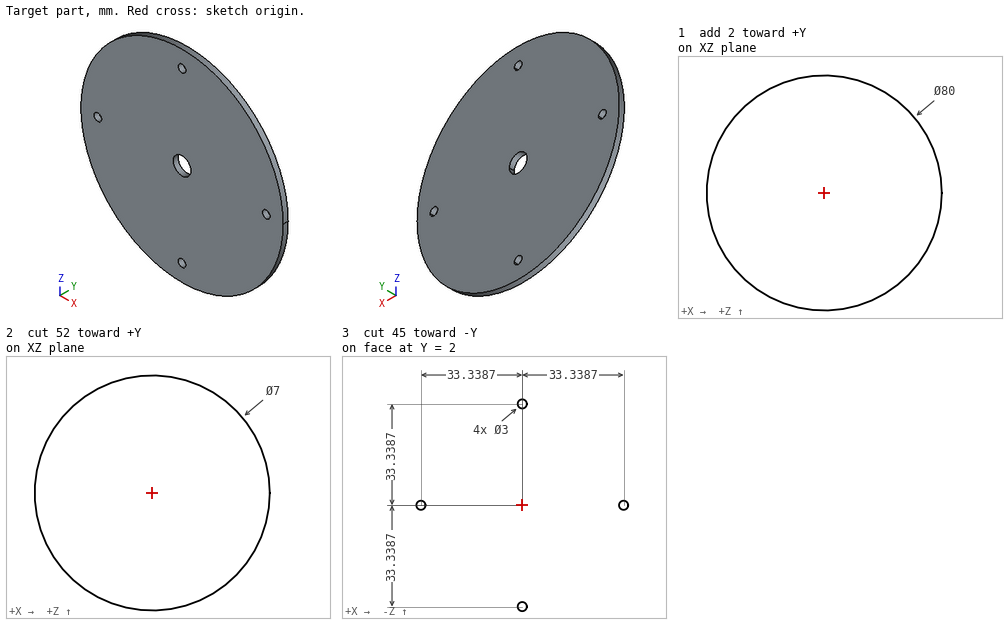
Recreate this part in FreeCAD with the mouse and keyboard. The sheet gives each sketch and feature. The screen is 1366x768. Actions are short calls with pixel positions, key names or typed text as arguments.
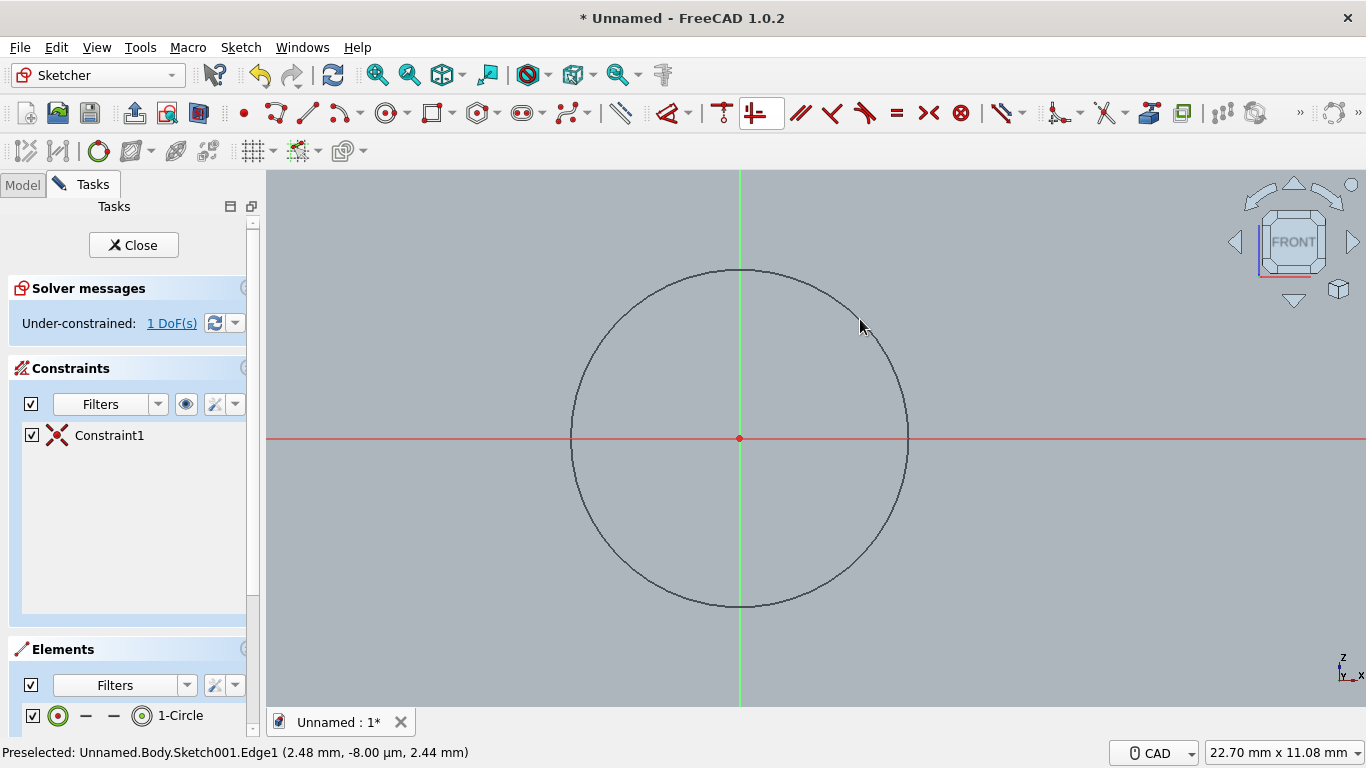
key(d)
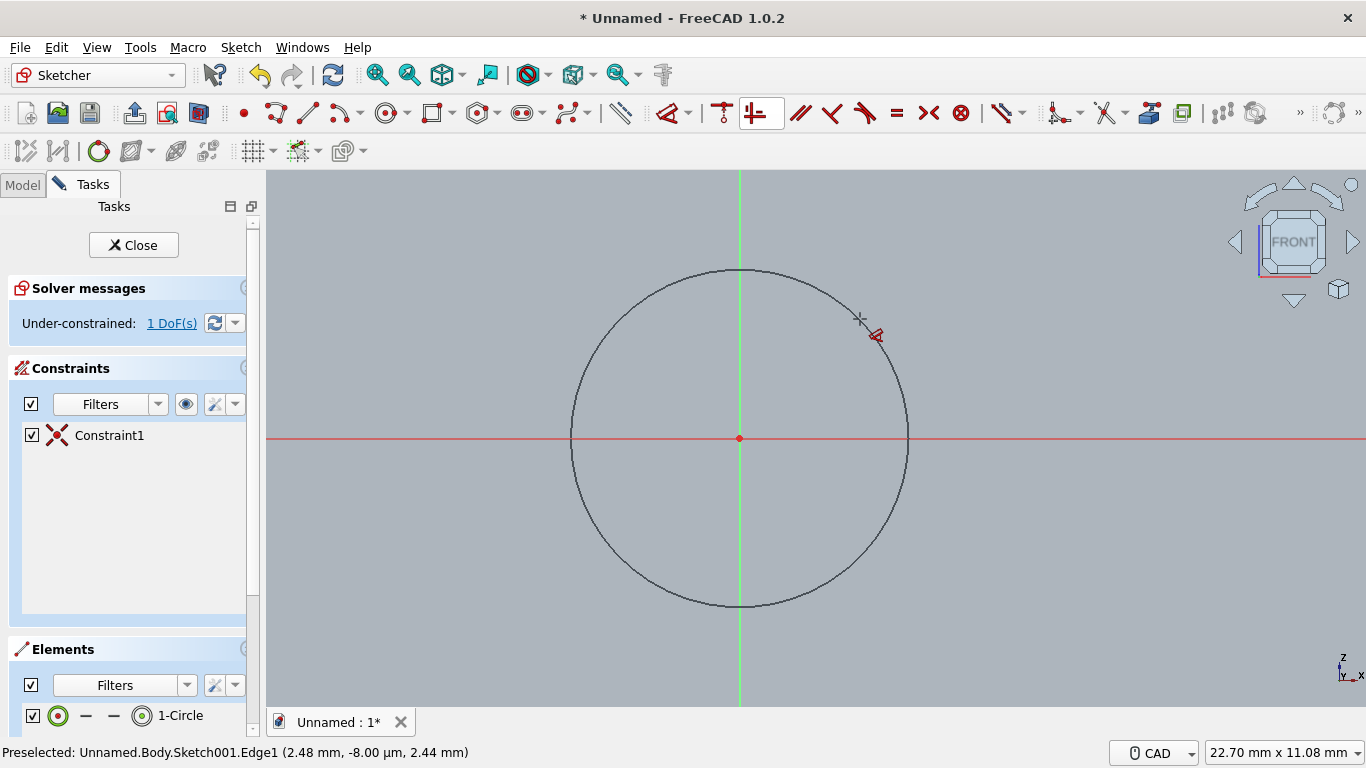
click(859, 319)
click(882, 296)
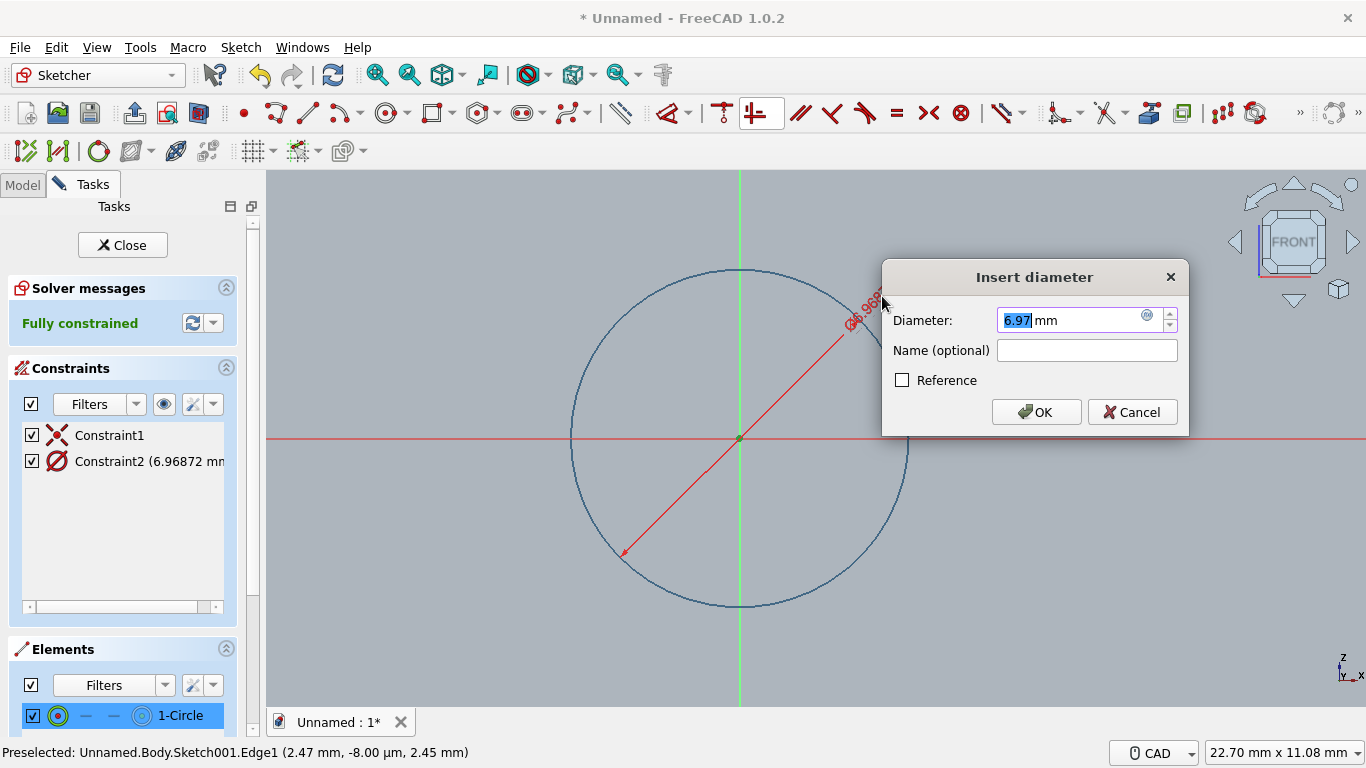
text(7)
key(Return)
key(Escape)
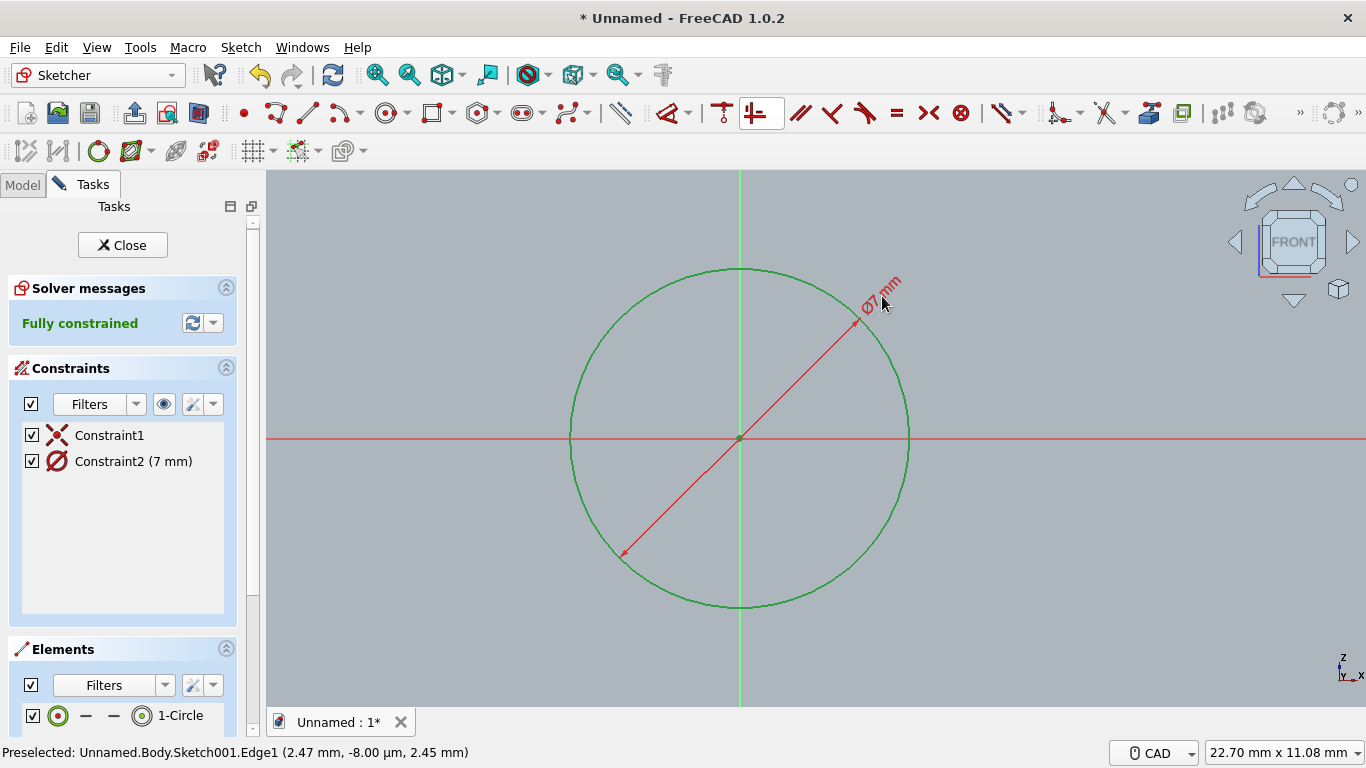
click(123, 245)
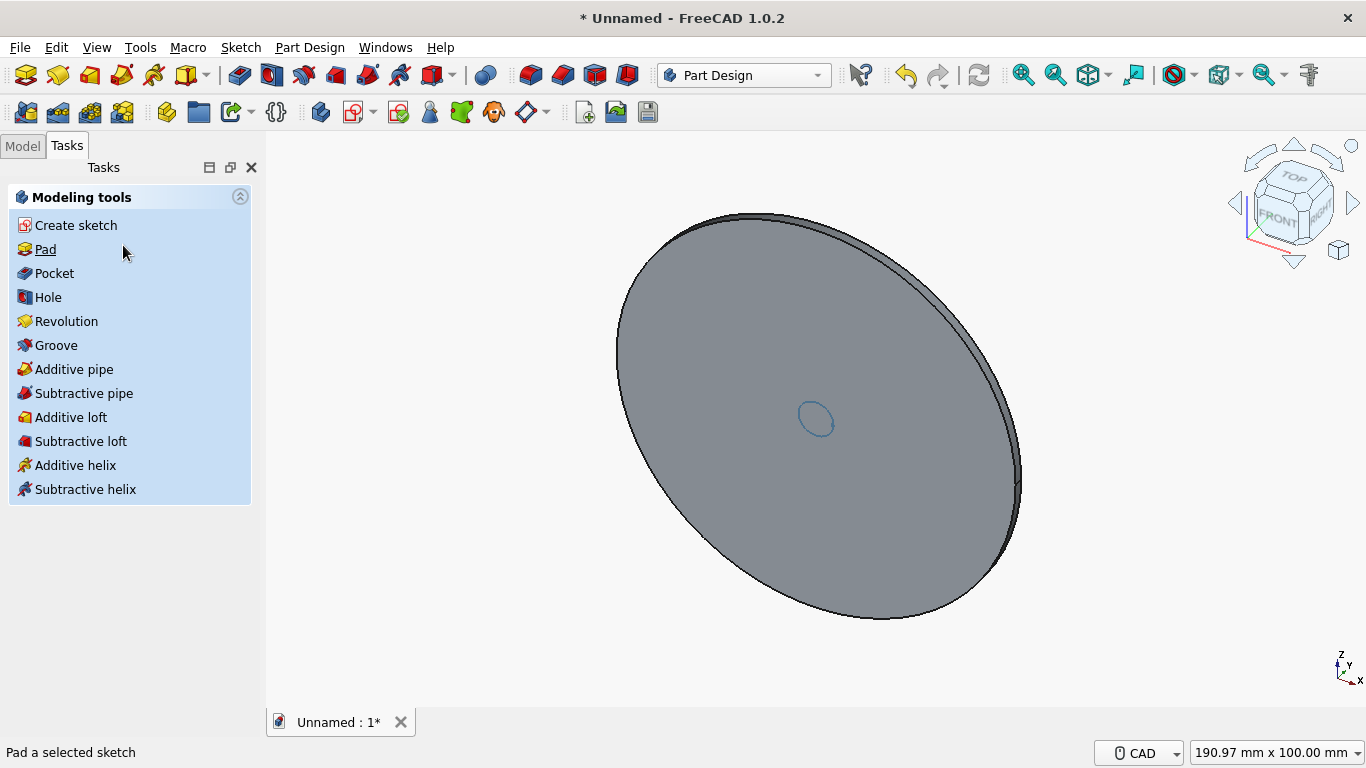
click(240, 76)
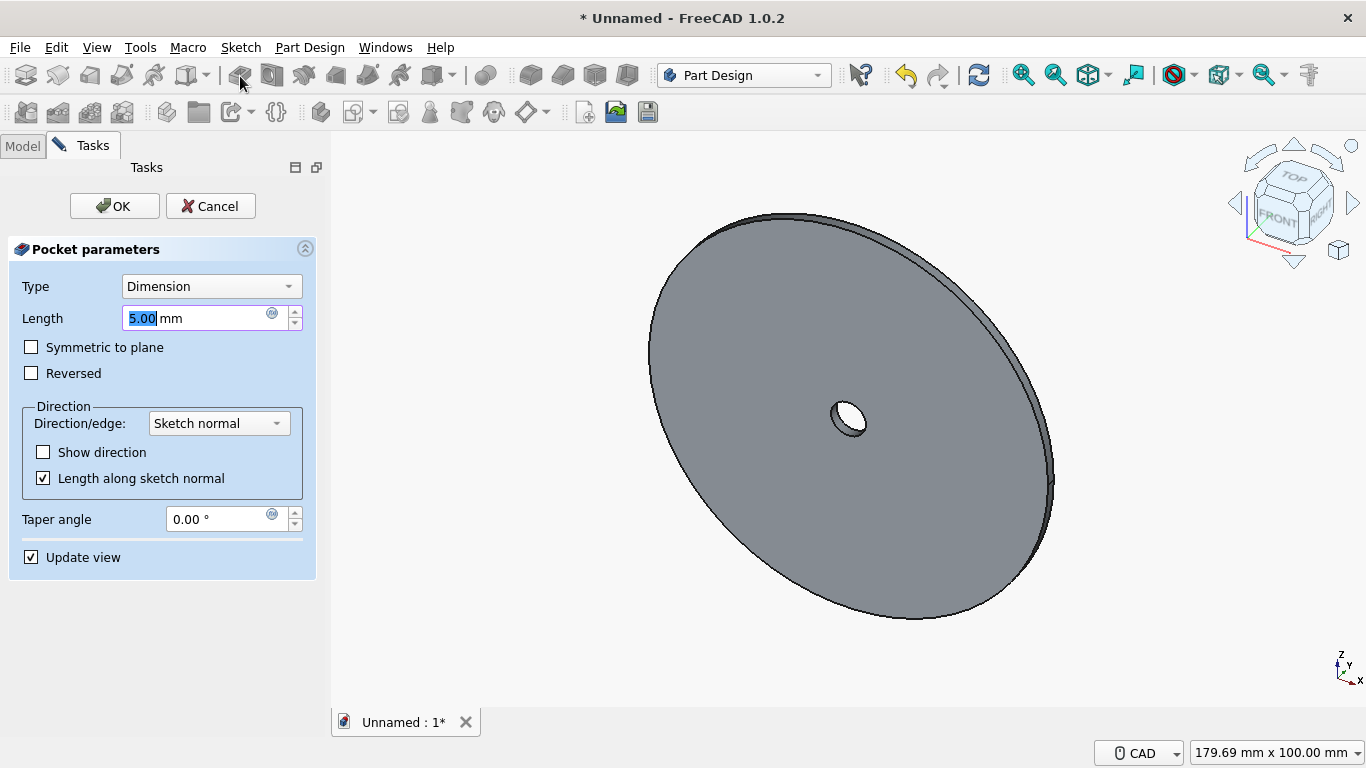
text(52)
key(Tab)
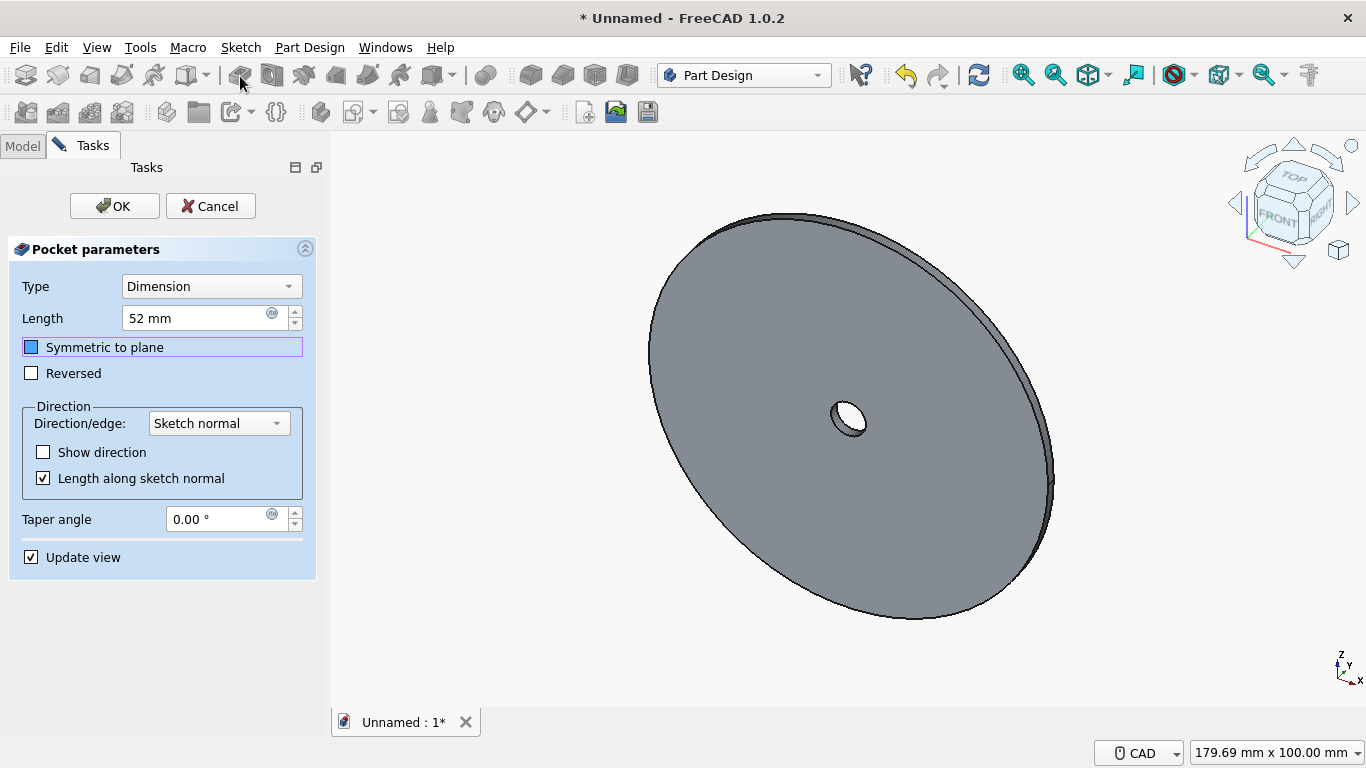
click(115, 206)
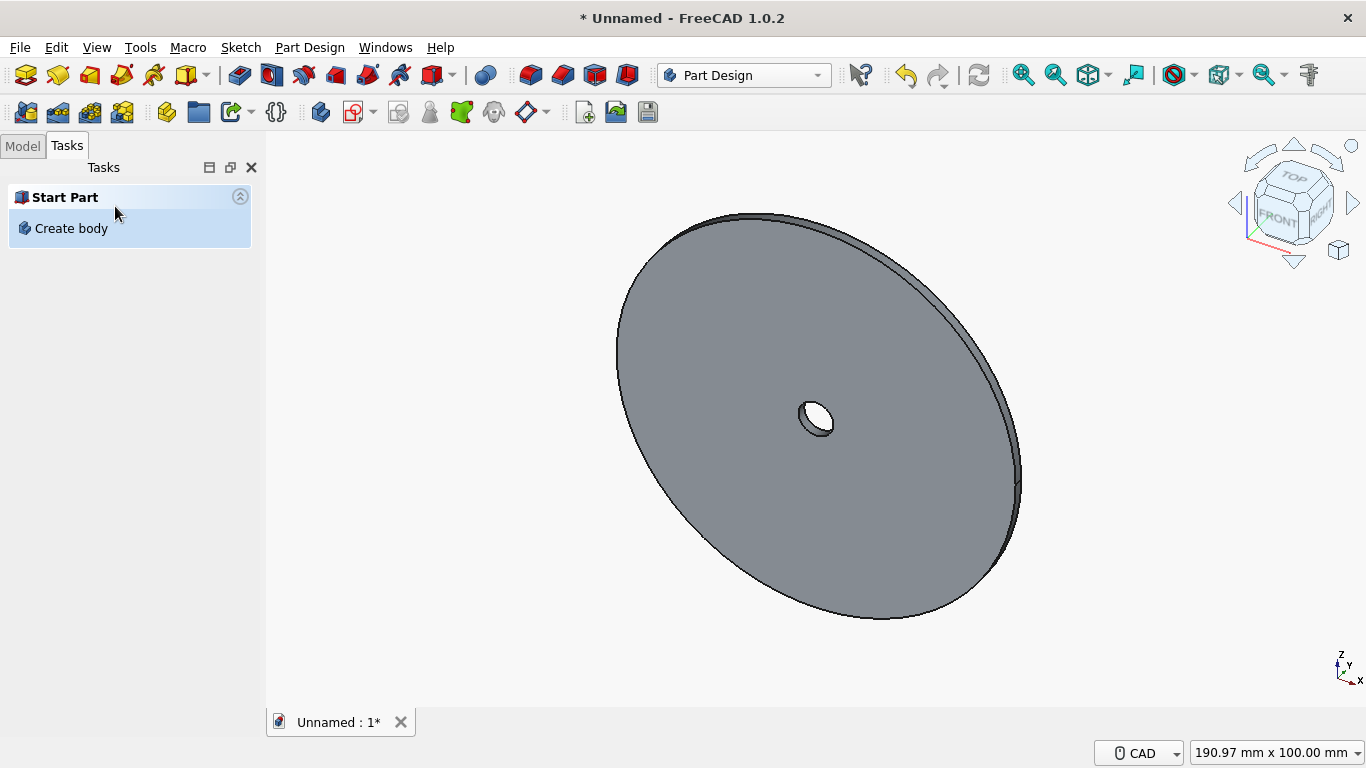
key(4)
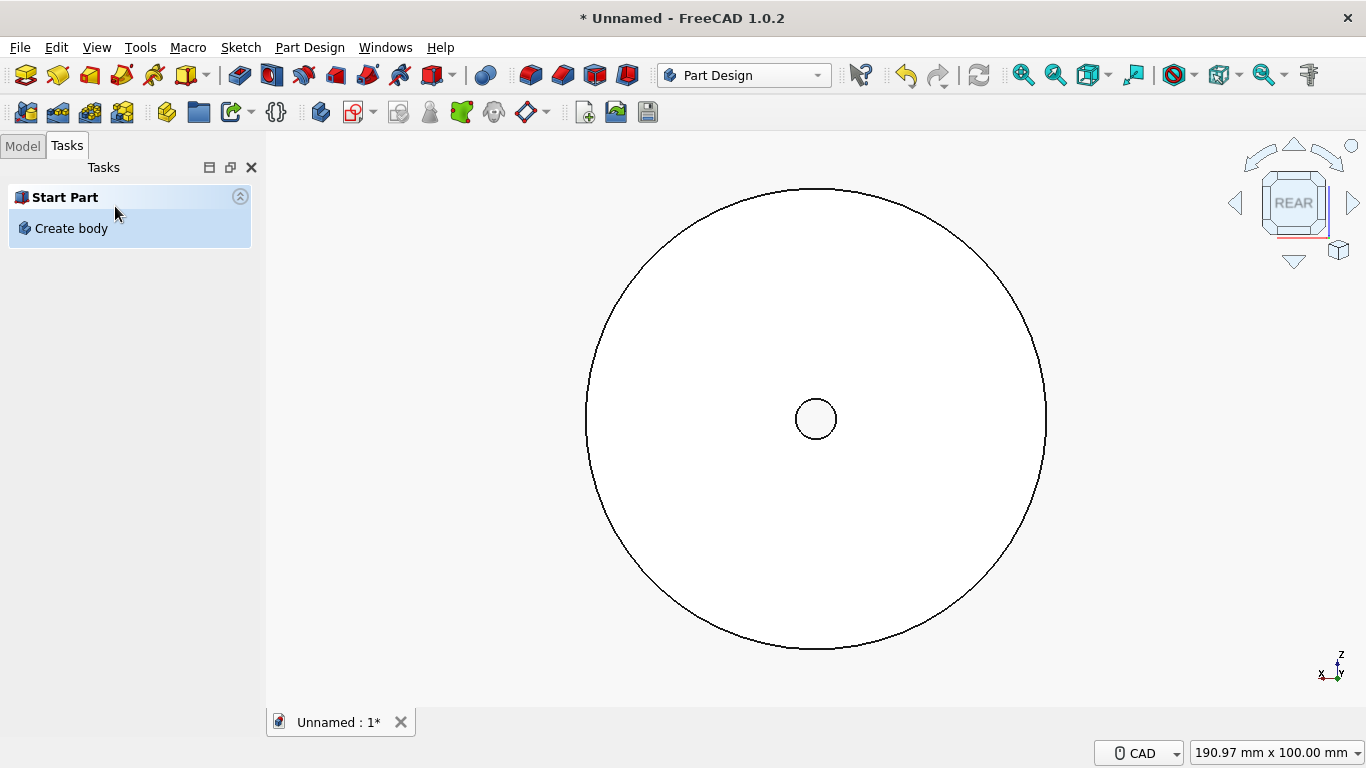
click(684, 418)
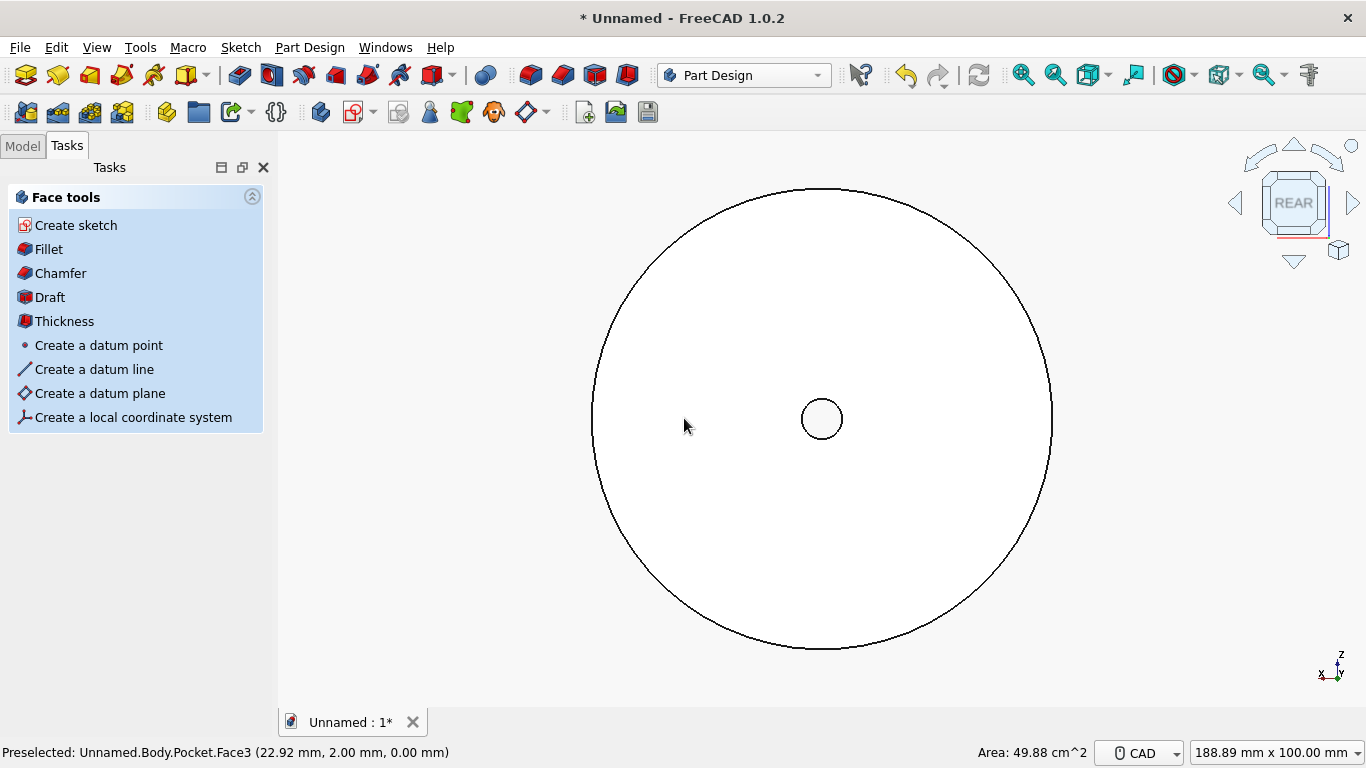
click(354, 112)